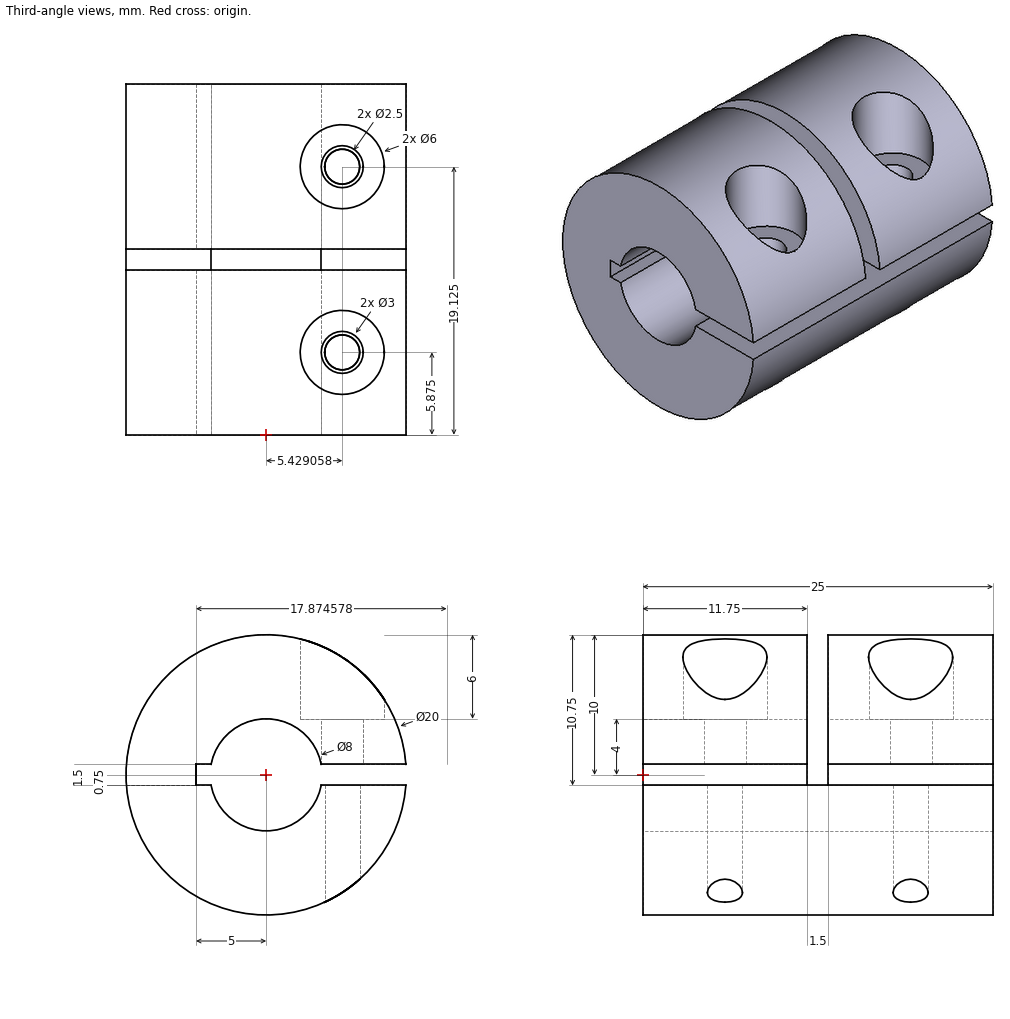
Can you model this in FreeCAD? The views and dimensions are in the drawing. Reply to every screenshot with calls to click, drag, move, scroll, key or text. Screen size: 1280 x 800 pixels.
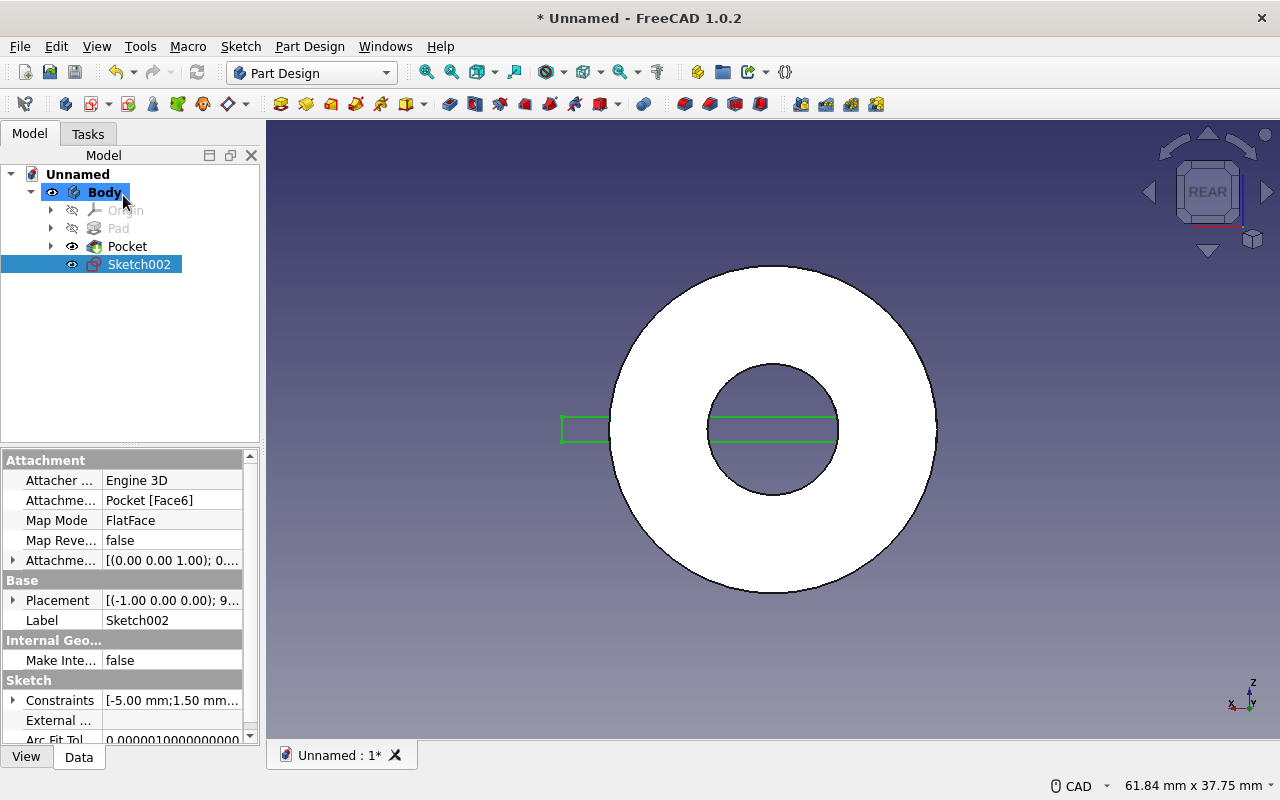
click(450, 104)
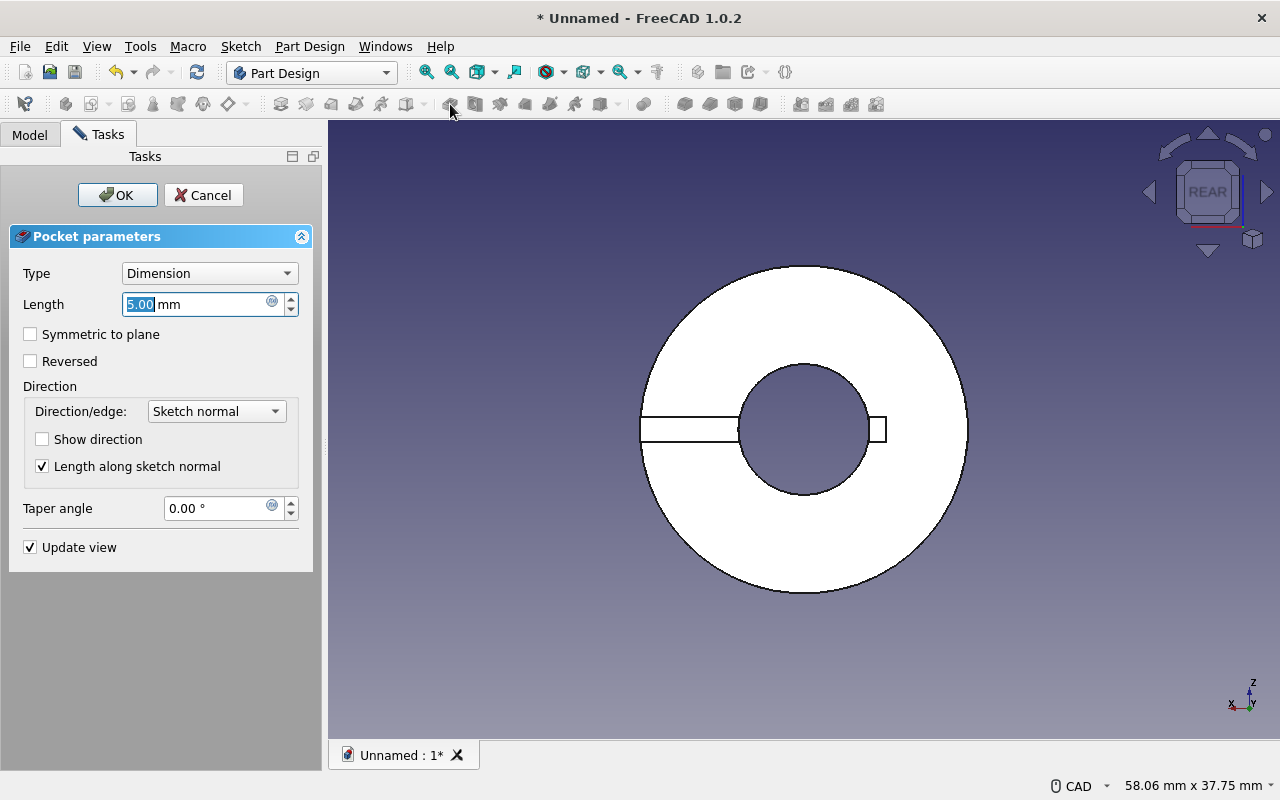
click(210, 274)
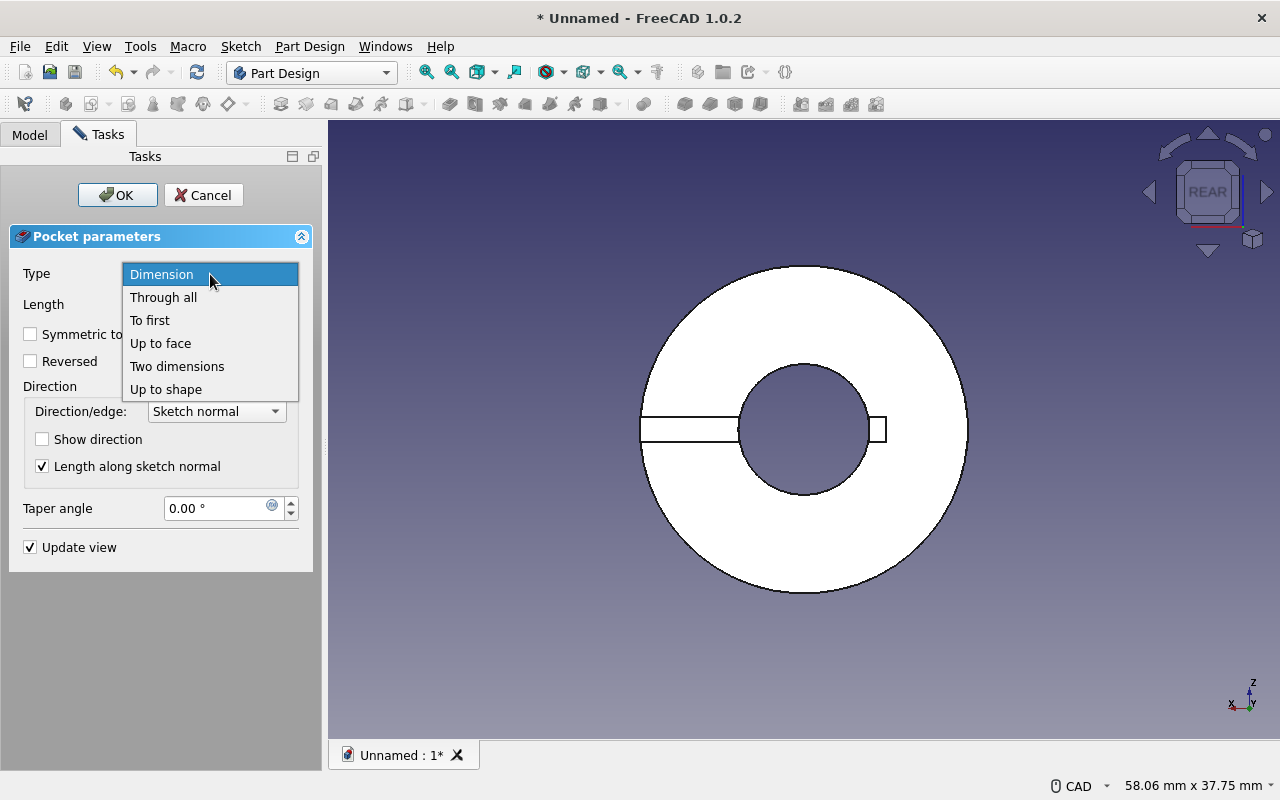
click(208, 298)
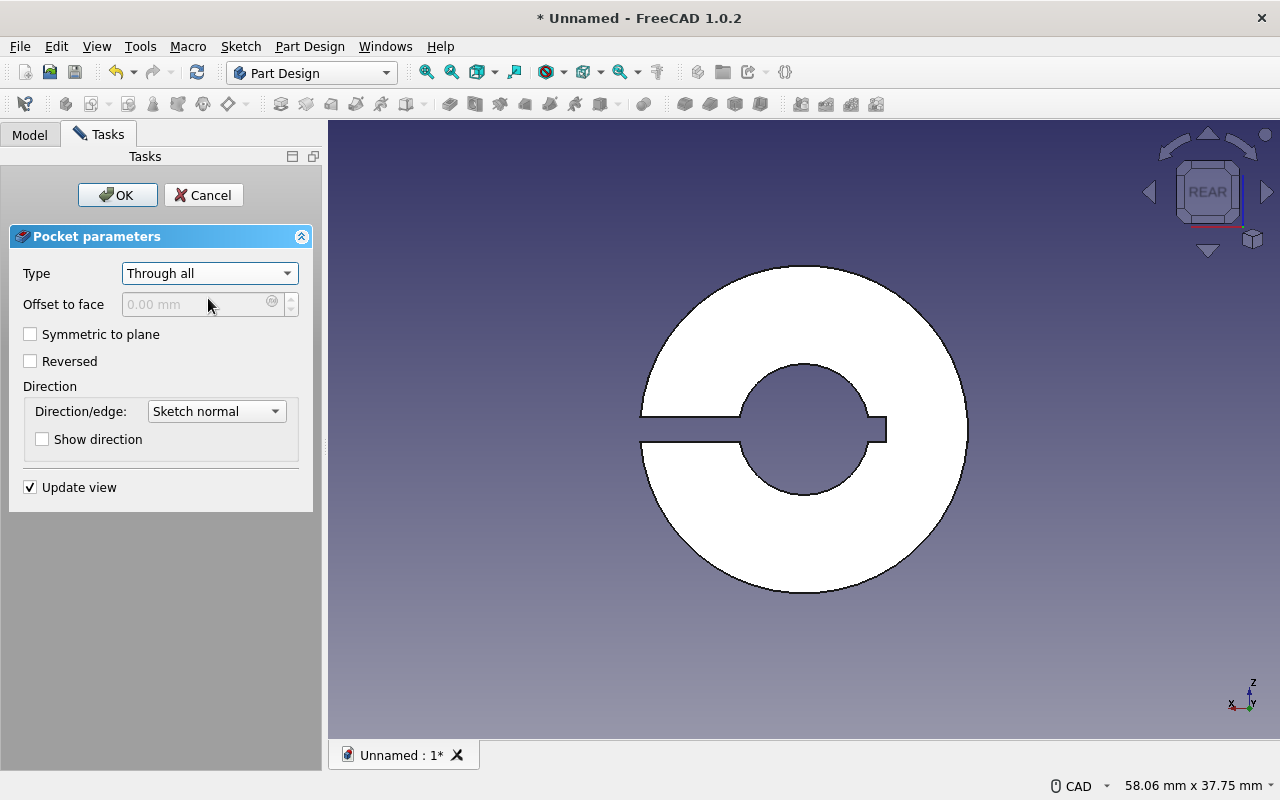
click(118, 195)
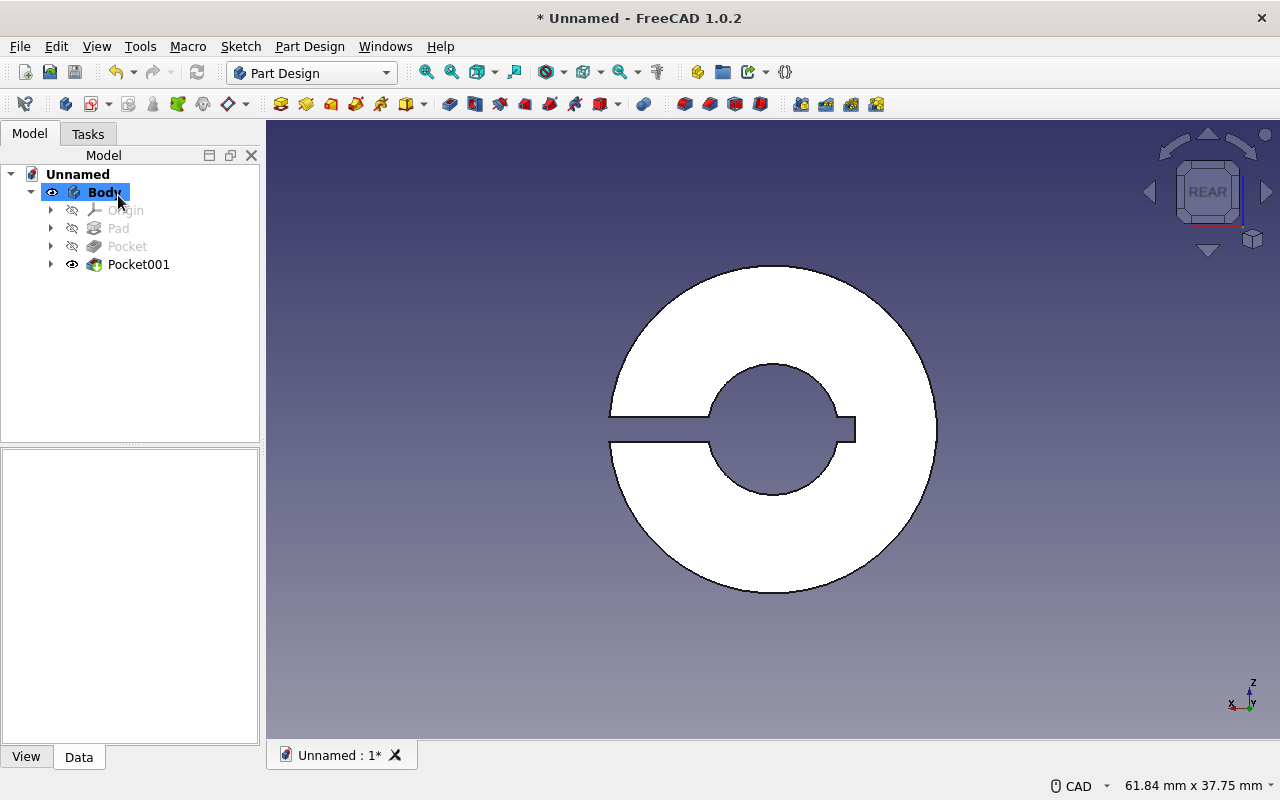
click(51, 210)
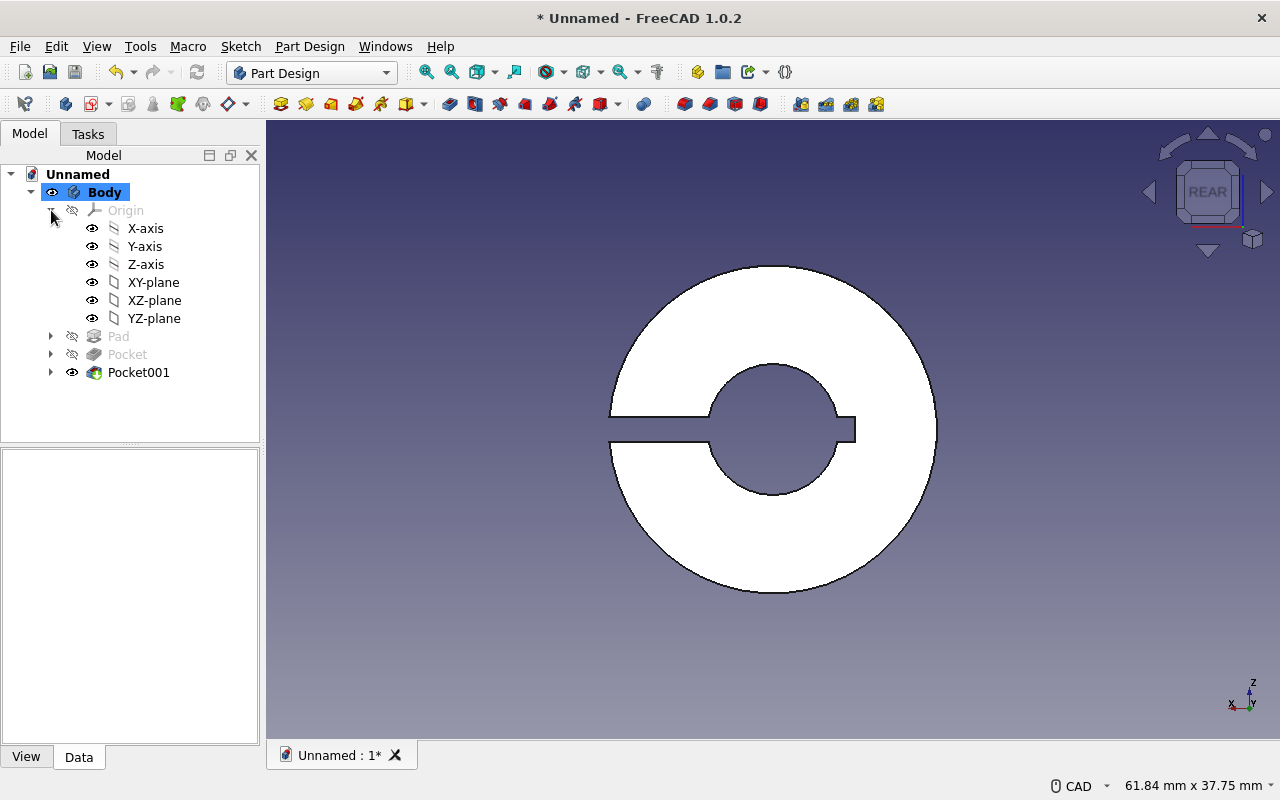
click(137, 282)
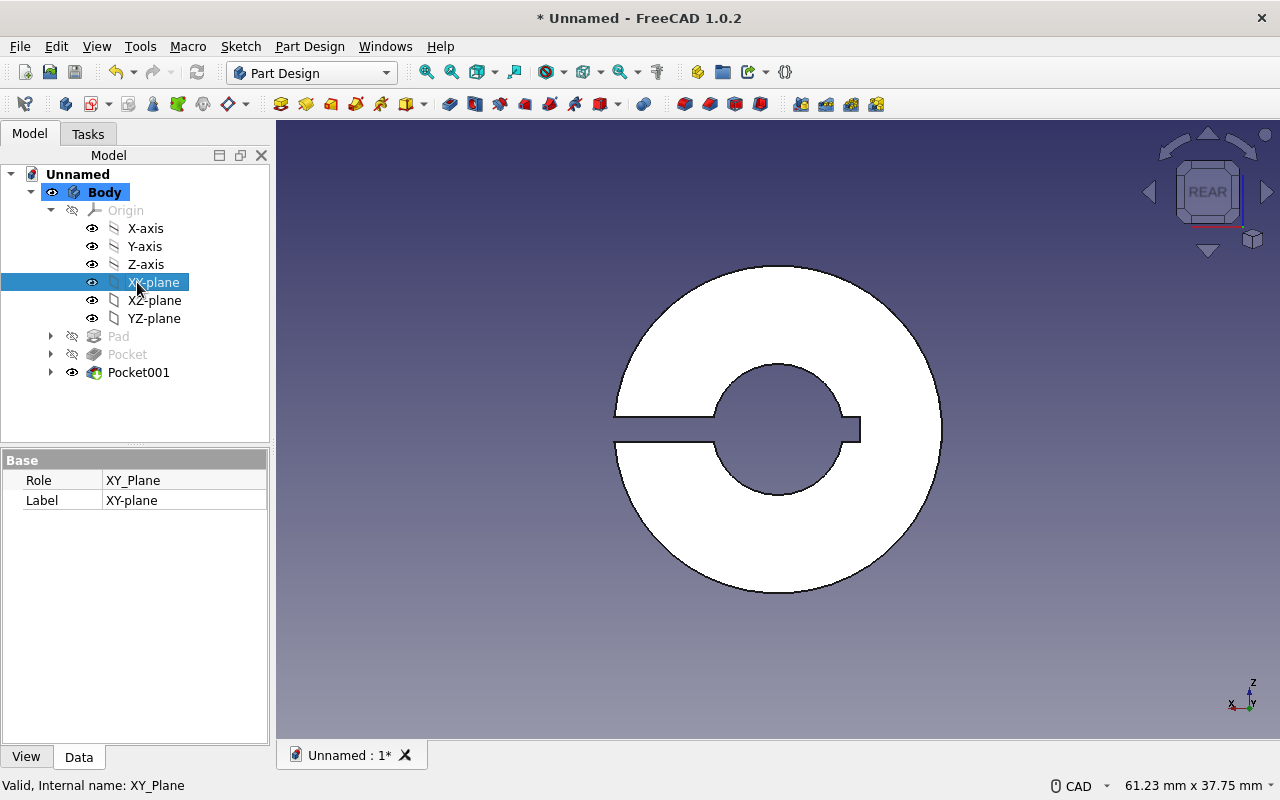
click(228, 104)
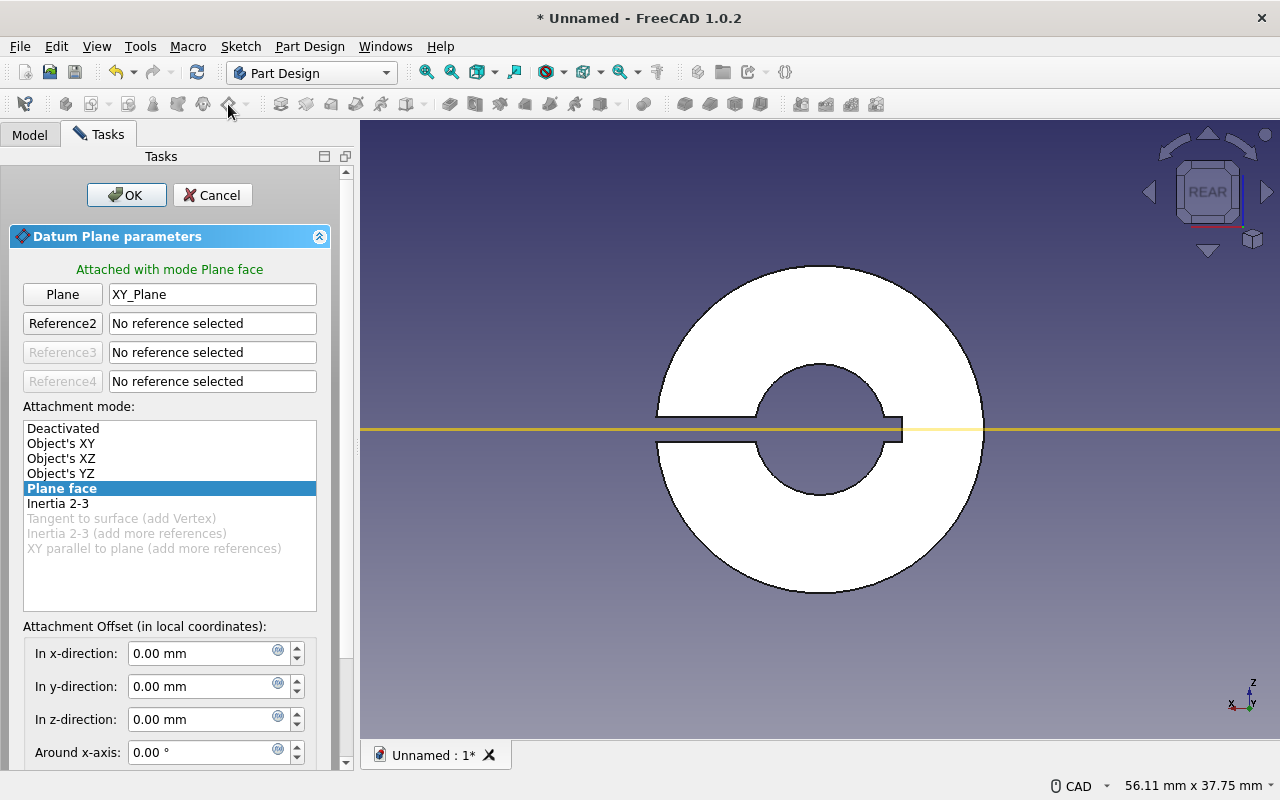
triple_click(210, 720)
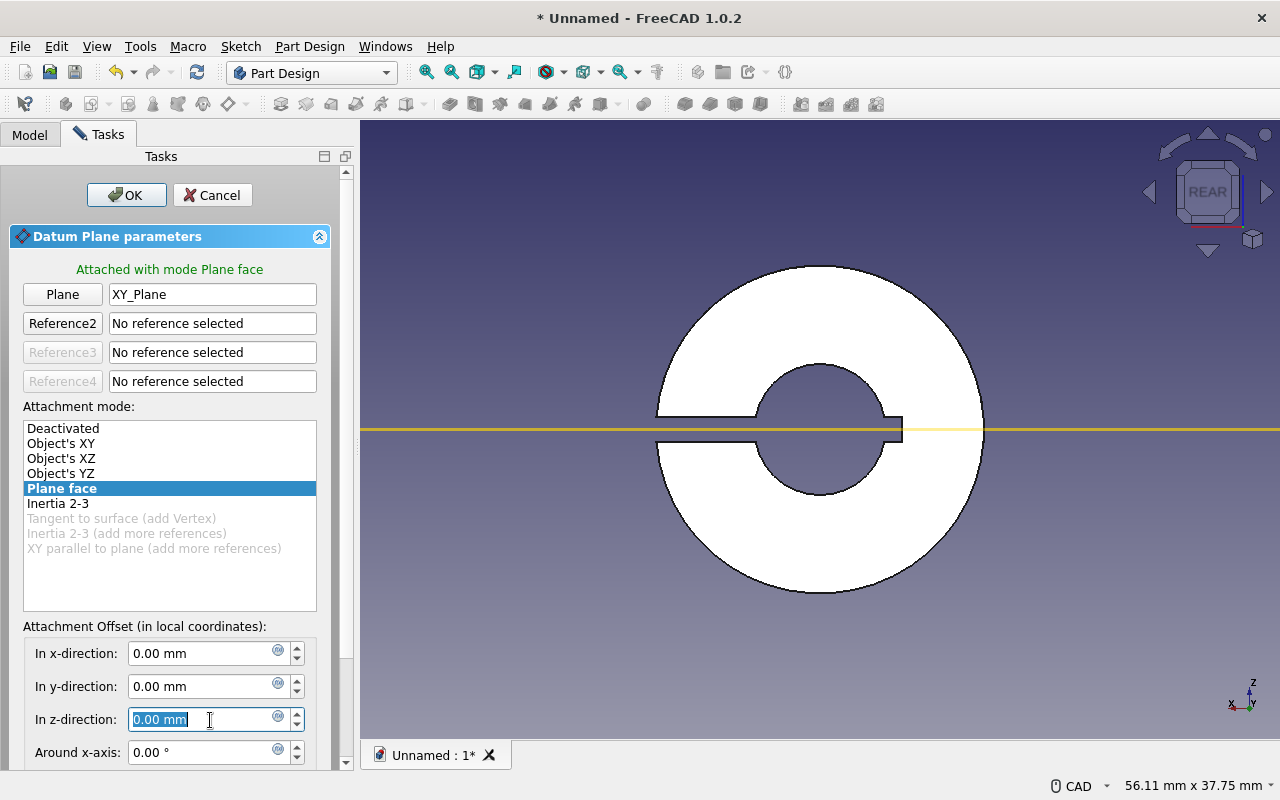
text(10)
key(Tab)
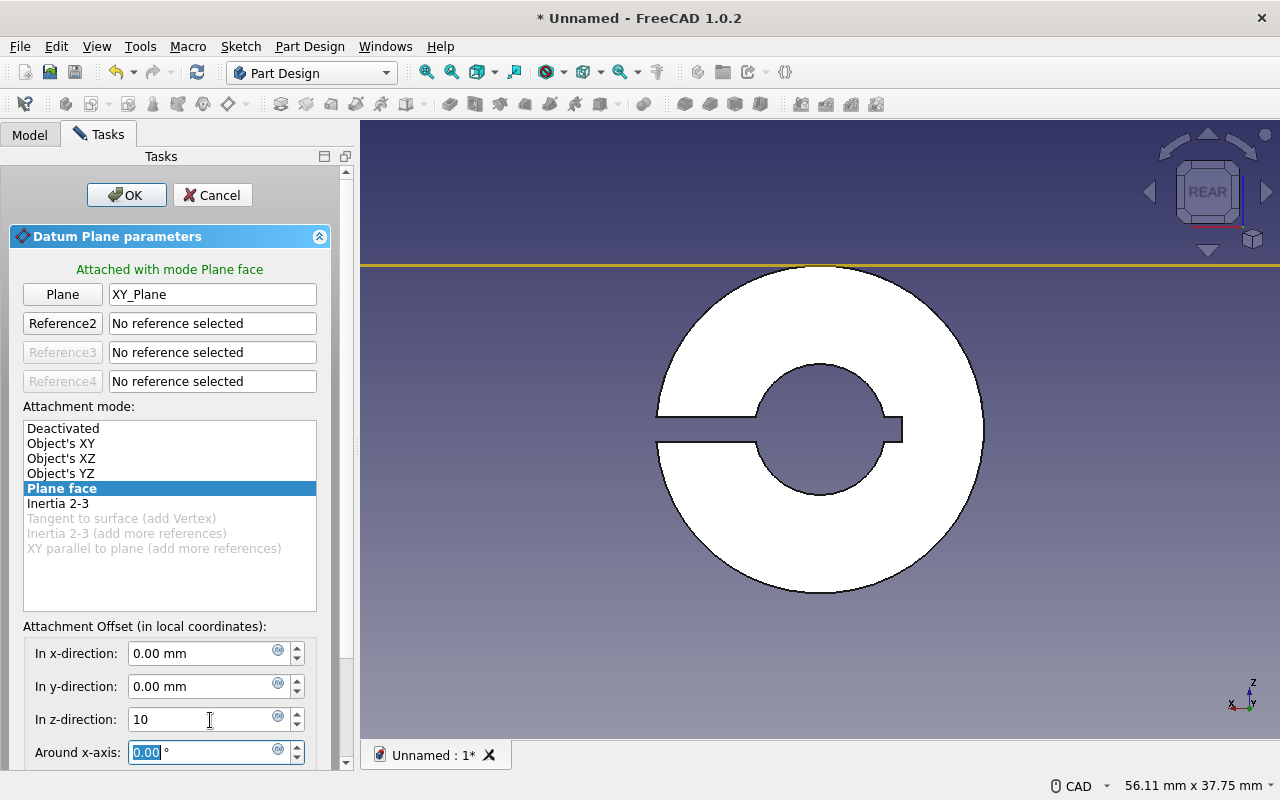
click(127, 195)